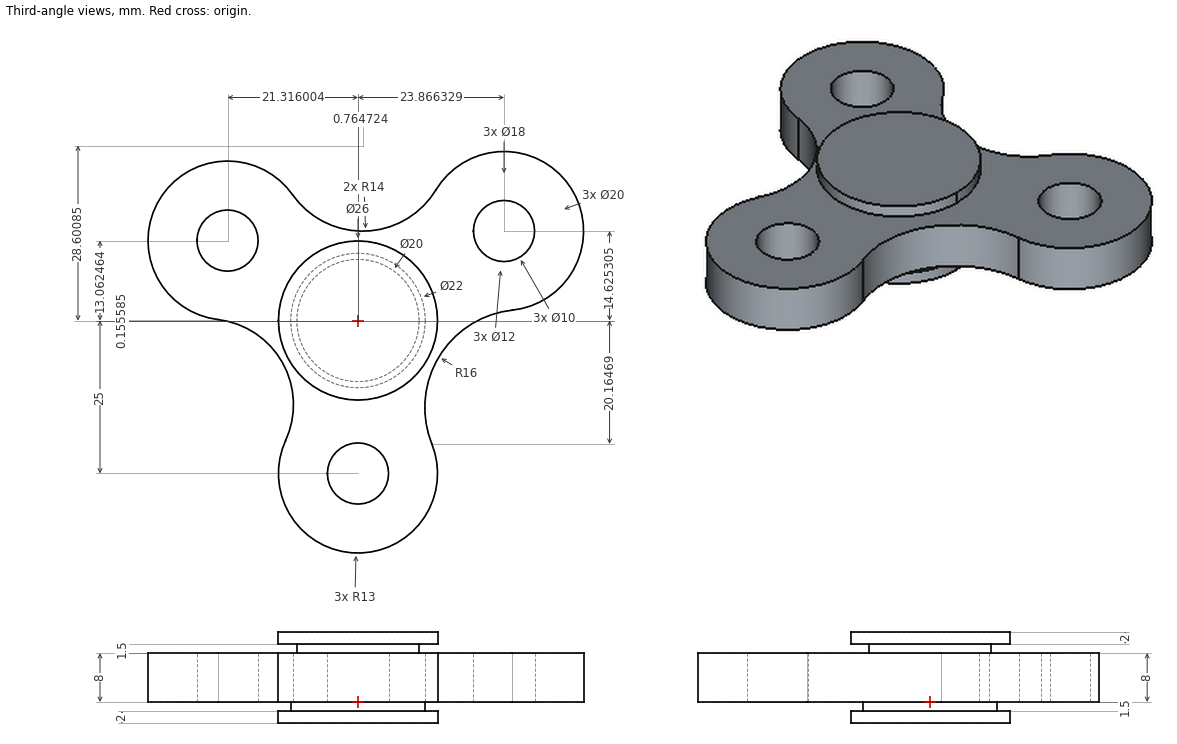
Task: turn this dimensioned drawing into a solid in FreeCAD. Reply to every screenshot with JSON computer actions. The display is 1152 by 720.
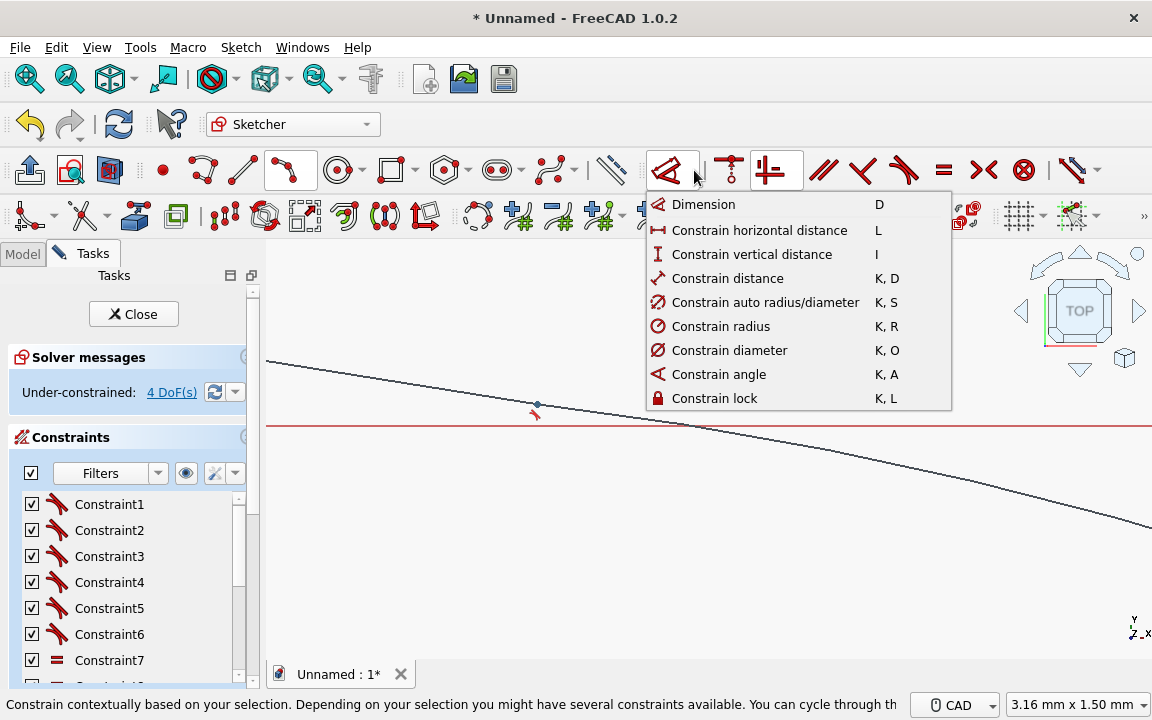
{"action": "left_click", "coordinate": [799, 254]}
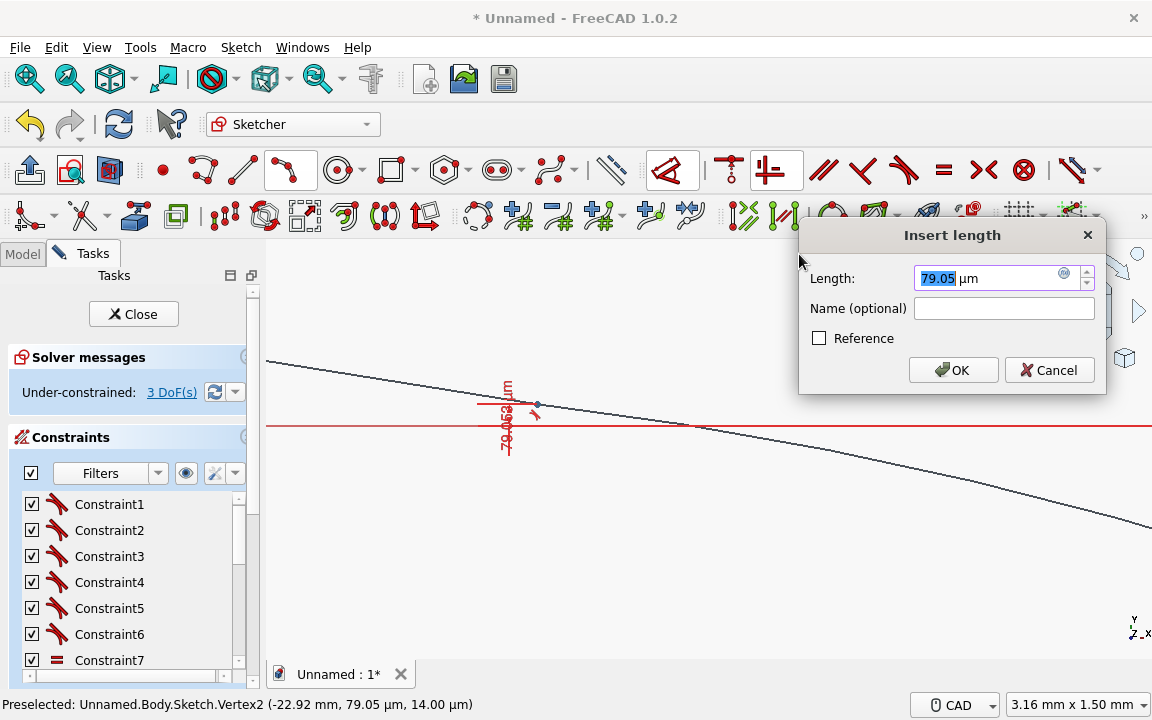
{"action": "key", "text": "ctrl+a"}
{"action": "type", "text": "0.155585 mm"}
{"action": "key", "text": "Return"}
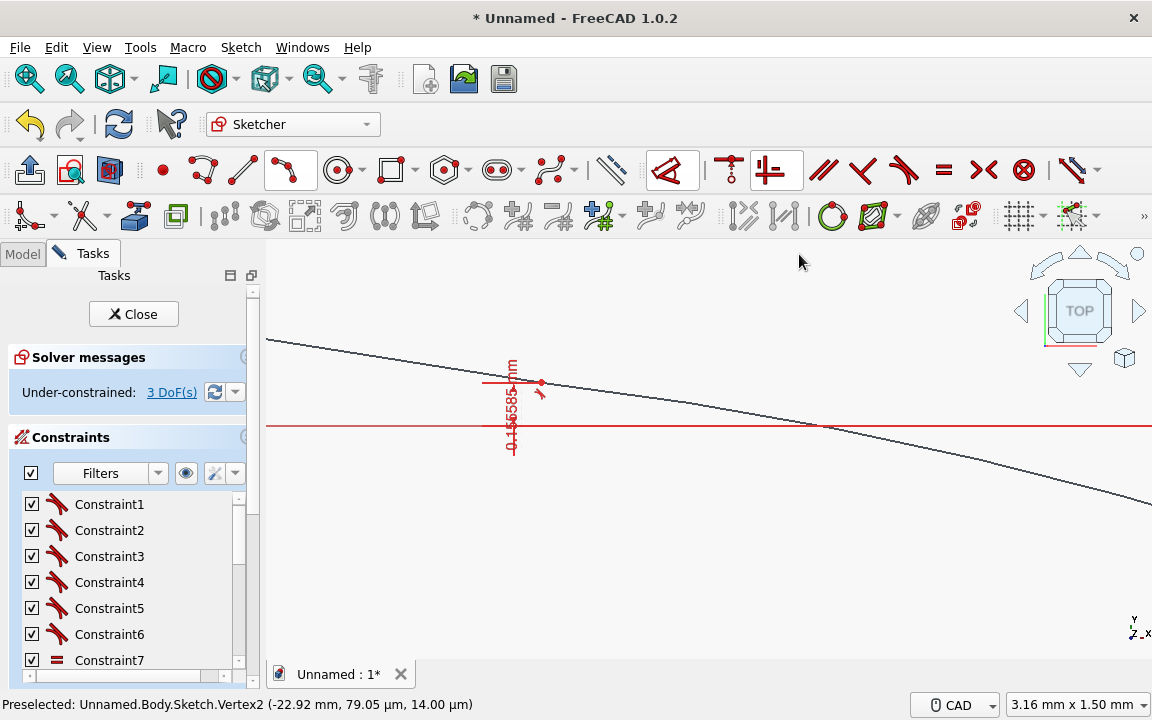
{"action": "scroll", "coordinate": [640, 449], "scroll_direction": "down", "scroll_amount": 15}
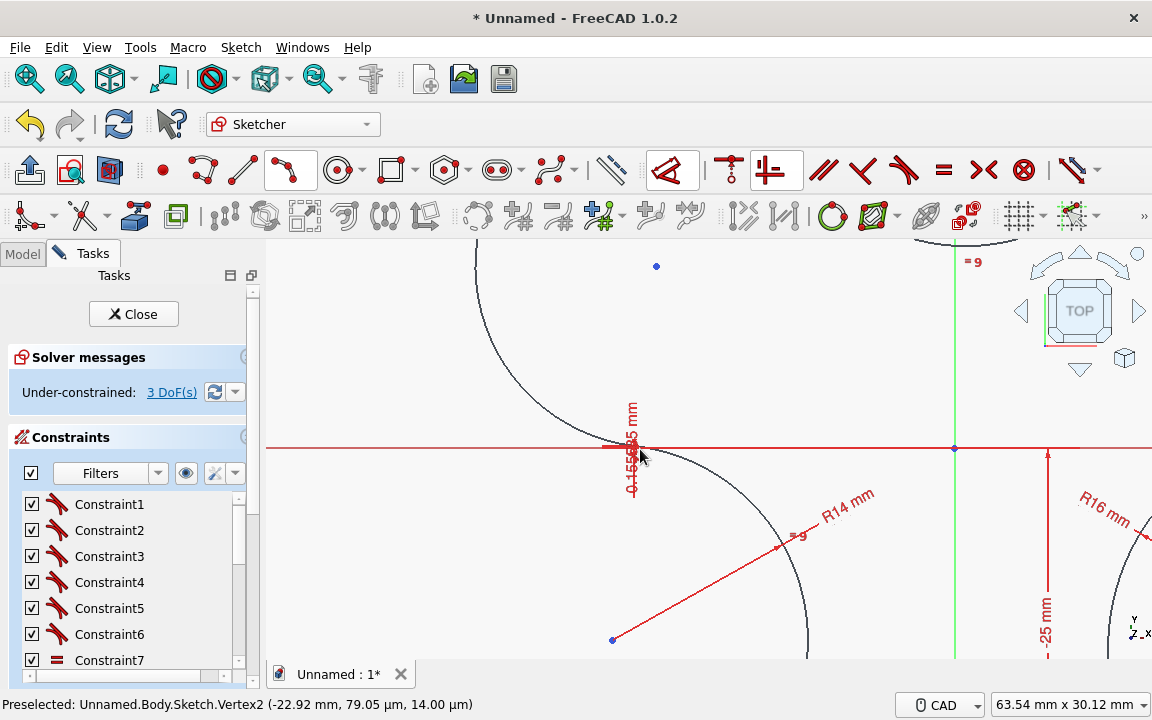
{"action": "scroll", "coordinate": [498, 400], "scroll_direction": "down", "scroll_amount": 6}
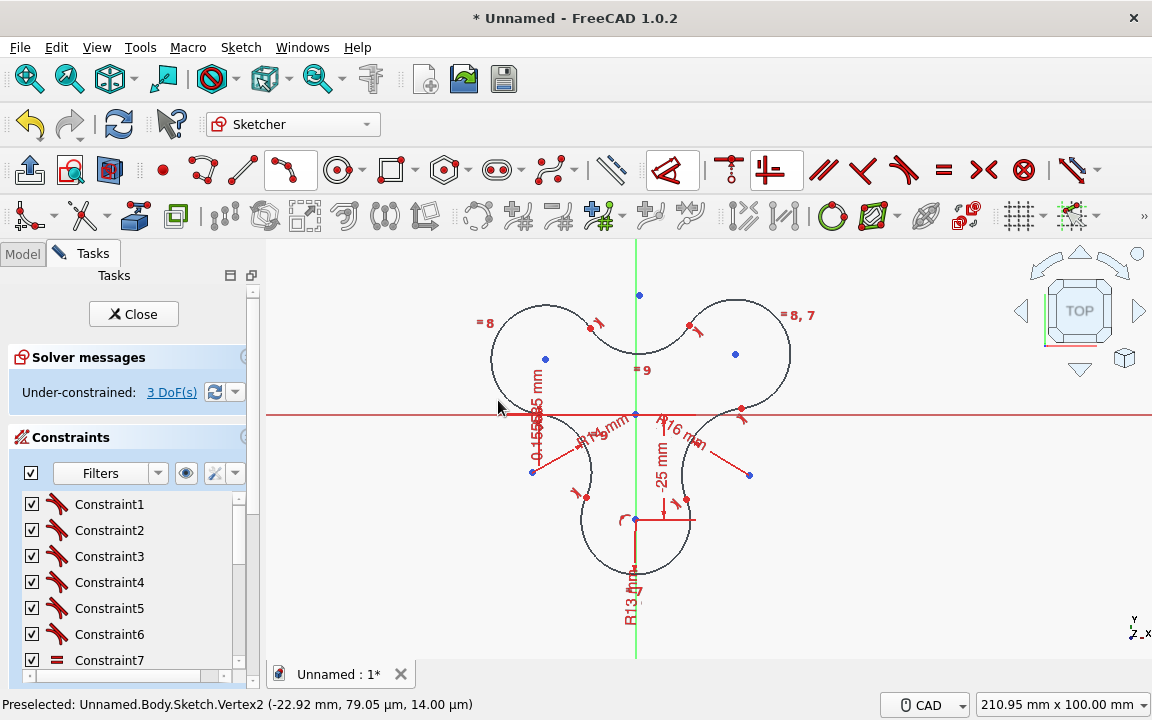
{"action": "left_click", "coordinate": [687, 500]}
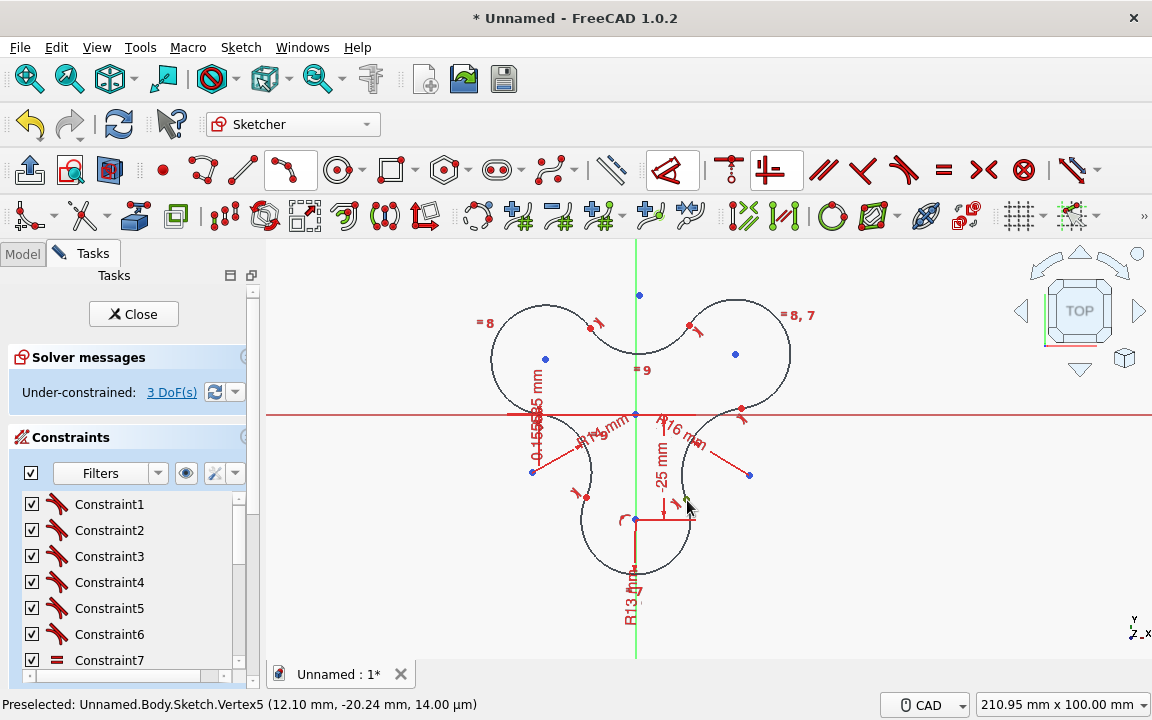
{"action": "left_click", "coordinate": [694, 170]}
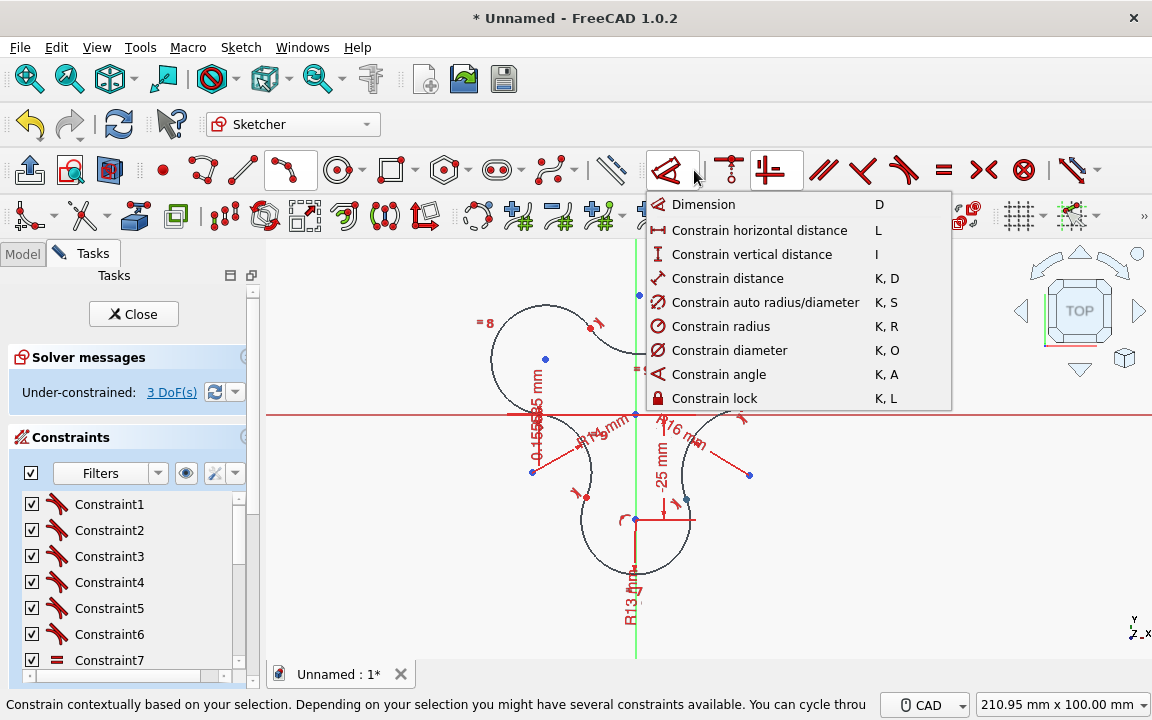
{"action": "left_click", "coordinate": [799, 254]}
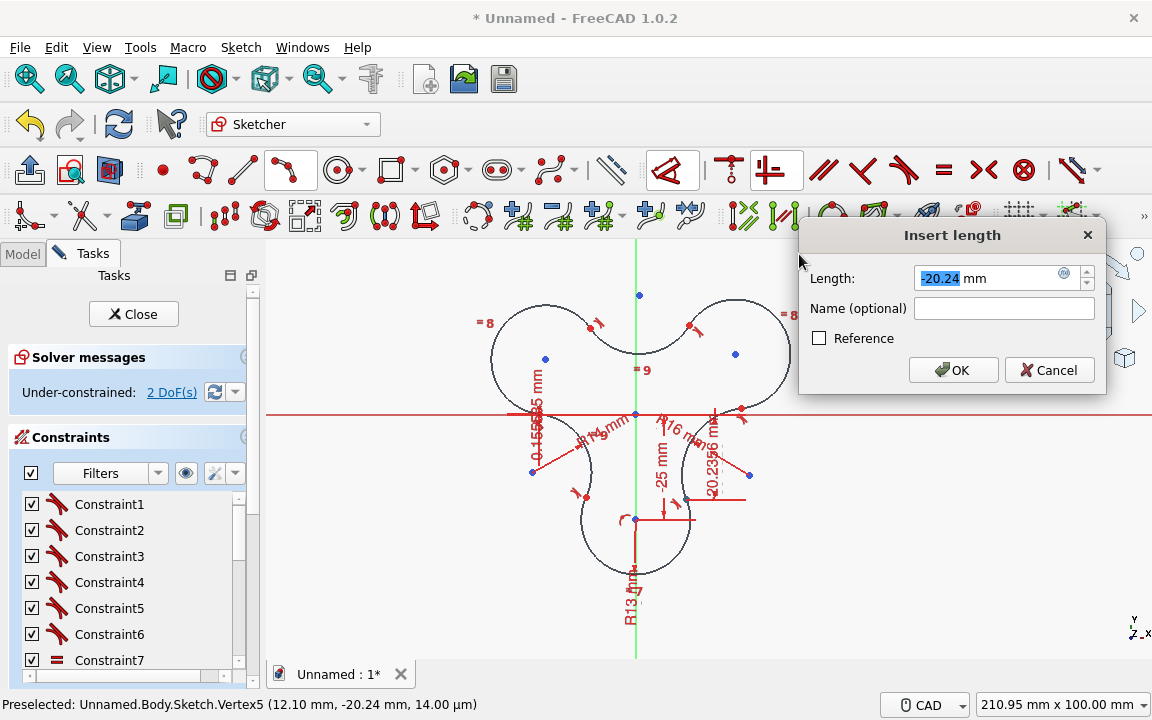
{"action": "type", "text": "-20.16469"}
{"action": "key", "text": "Return"}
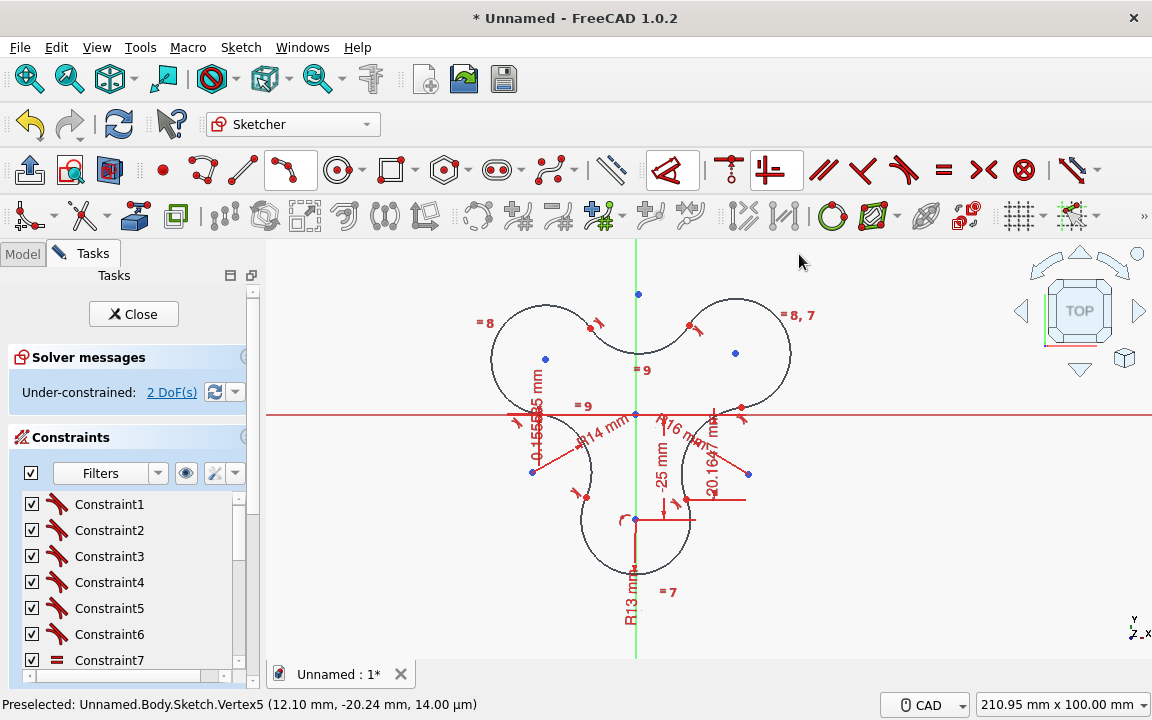
{"action": "scroll", "coordinate": [639, 295], "scroll_direction": "up", "scroll_amount": 13}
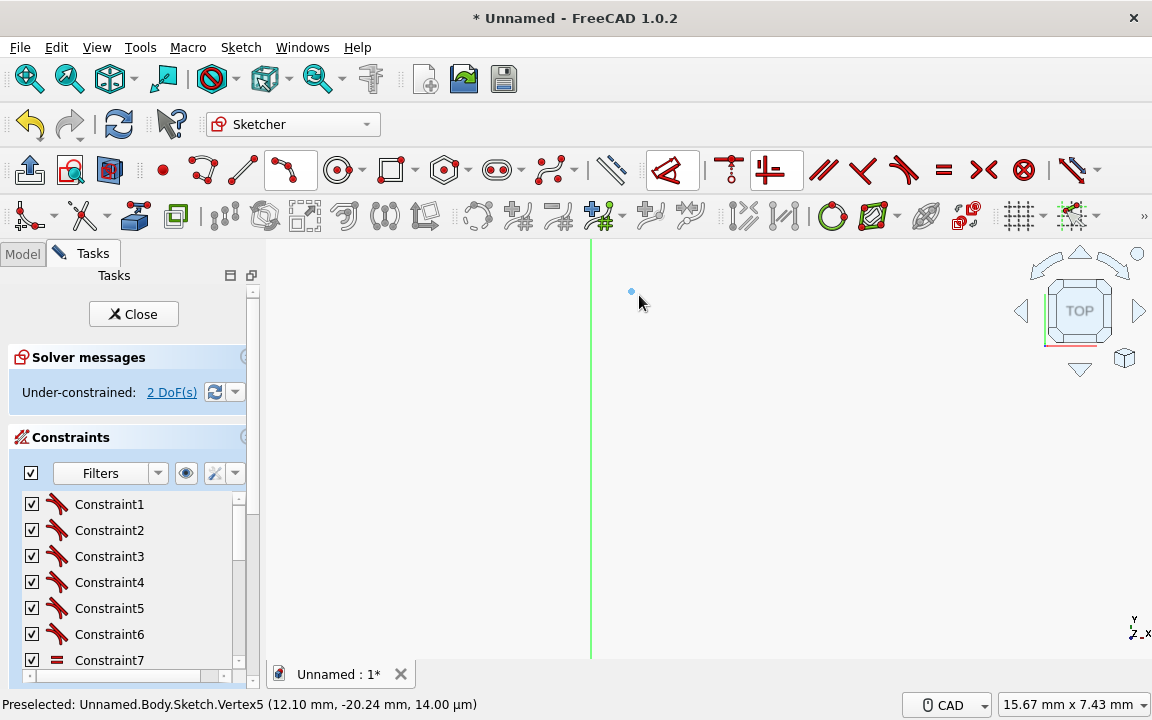
{"action": "left_click", "coordinate": [632, 292]}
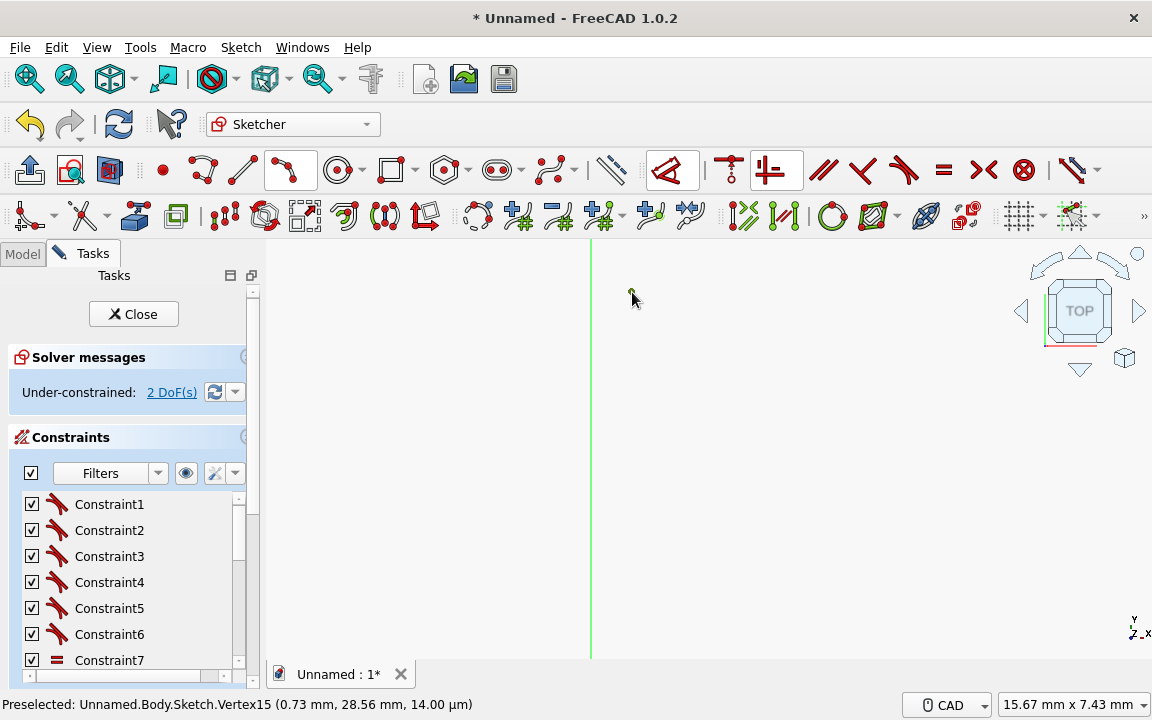
{"action": "left_click", "coordinate": [694, 170]}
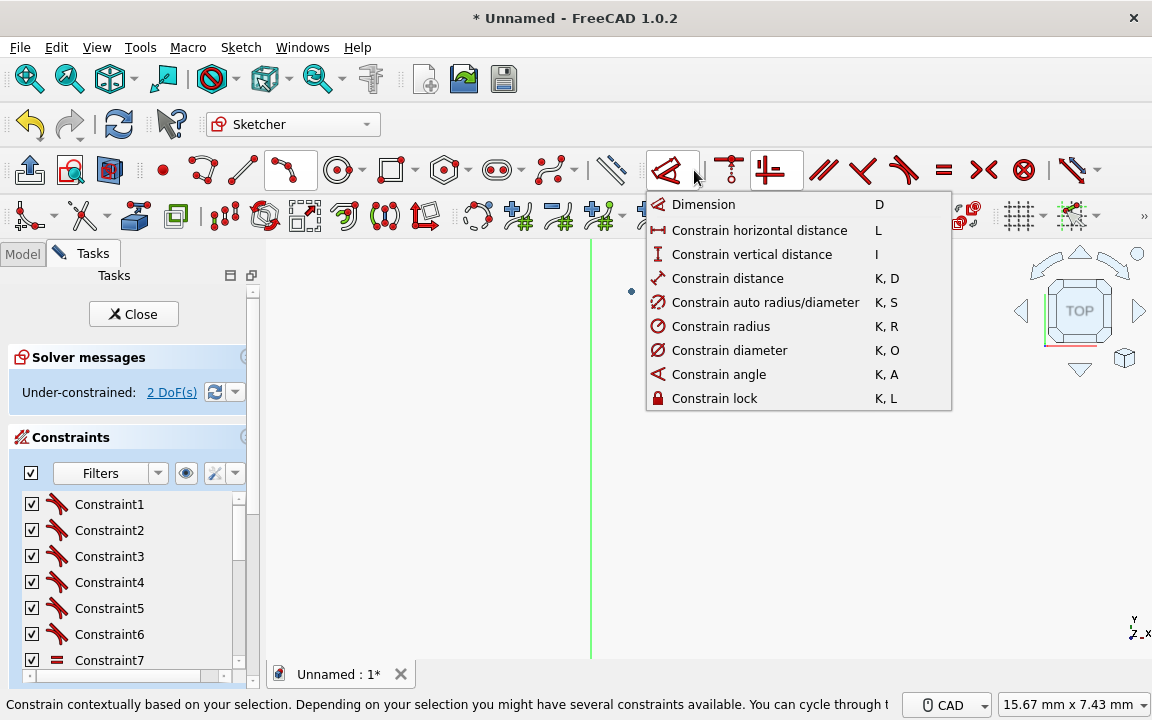
{"action": "left_click", "coordinate": [799, 230]}